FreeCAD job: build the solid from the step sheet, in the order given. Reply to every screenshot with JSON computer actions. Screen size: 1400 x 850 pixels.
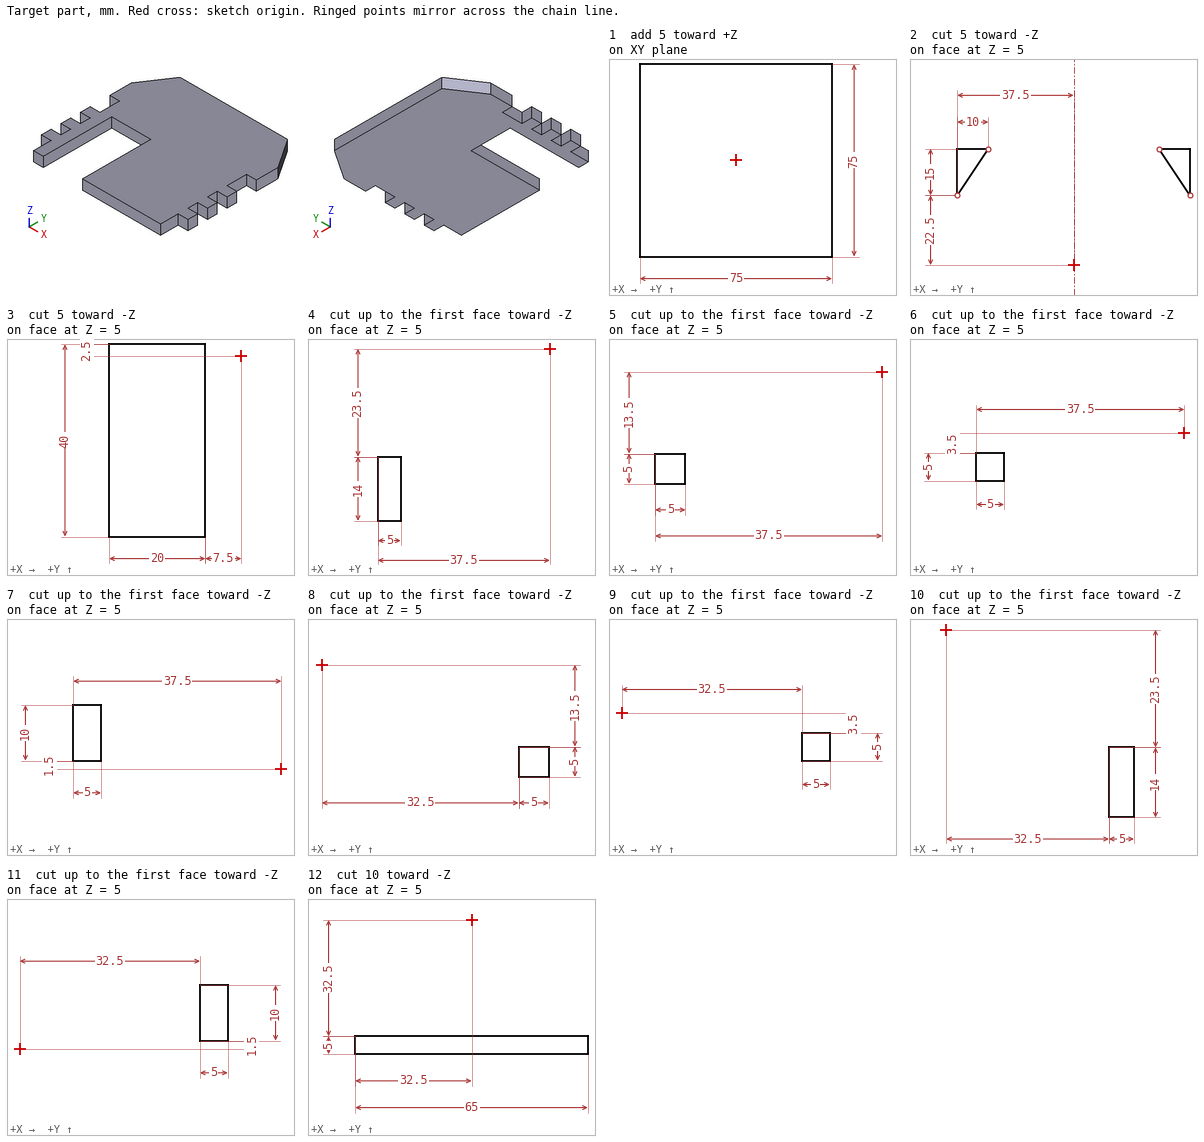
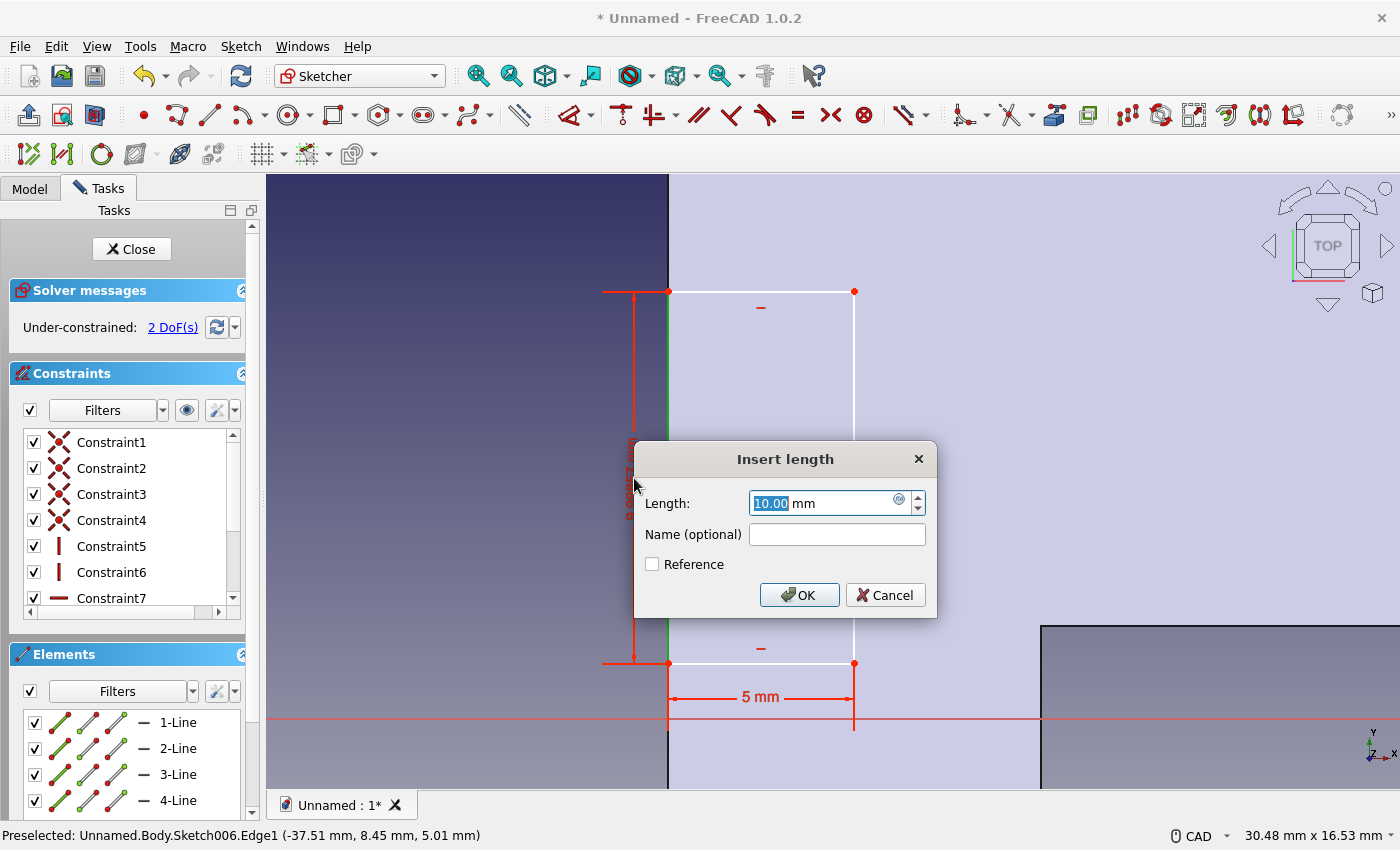
{"action": "type", "text": "10"}
{"action": "key", "text": "Return"}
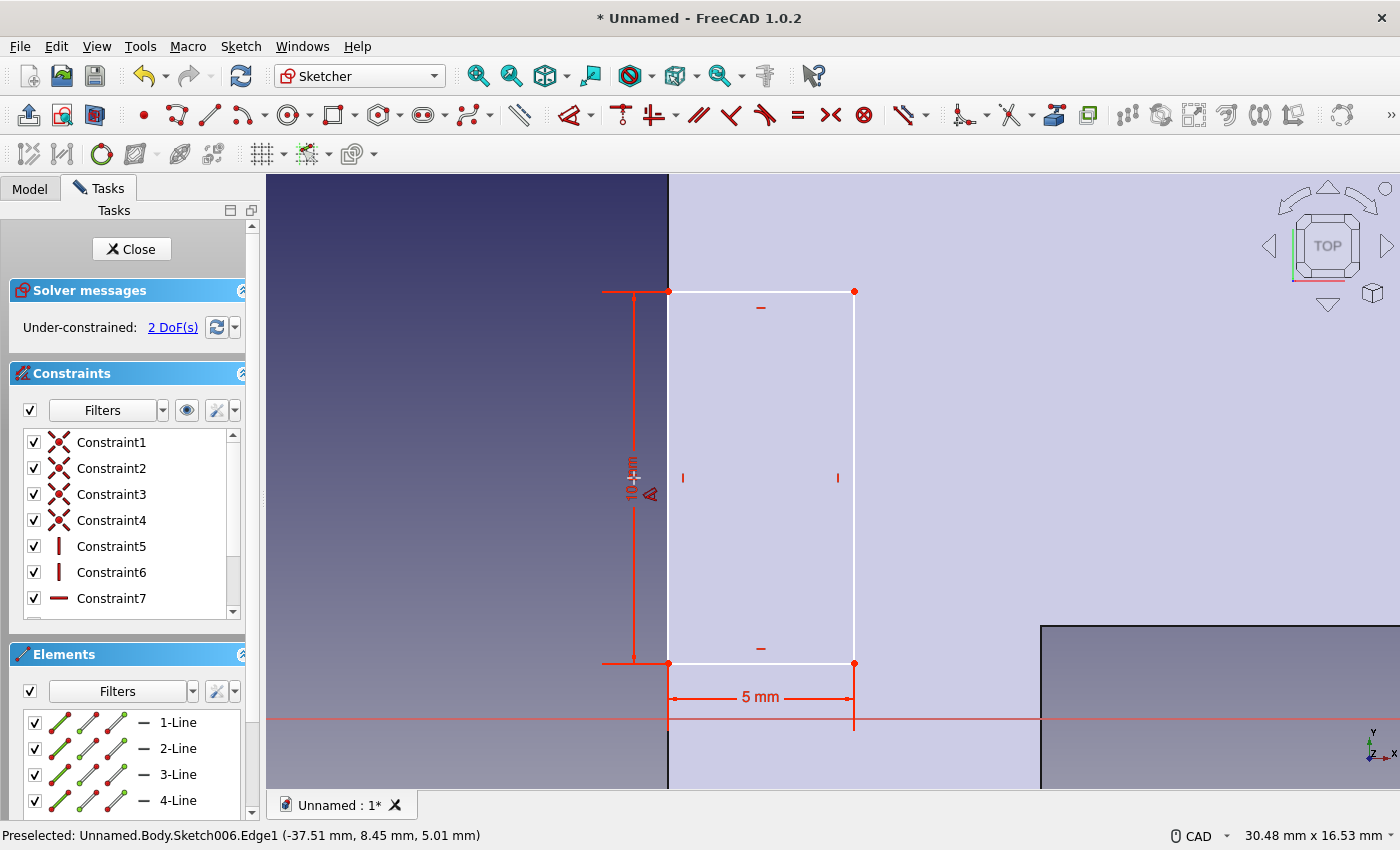
{"action": "left_click", "coordinate": [668, 664]}
{"action": "left_click", "coordinate": [634, 692]}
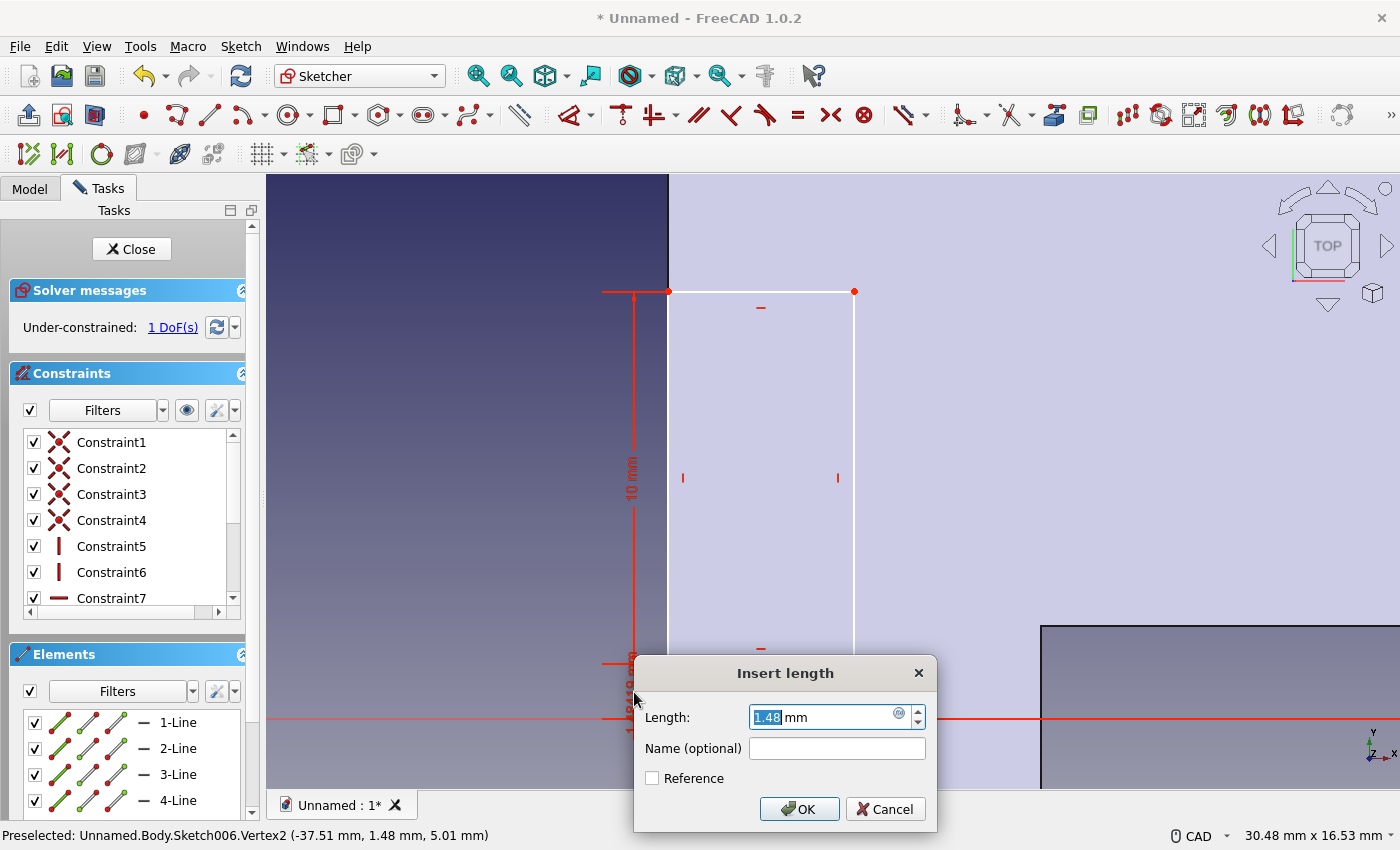
{"action": "type", "text": "1.5"}
{"action": "key", "text": "Return"}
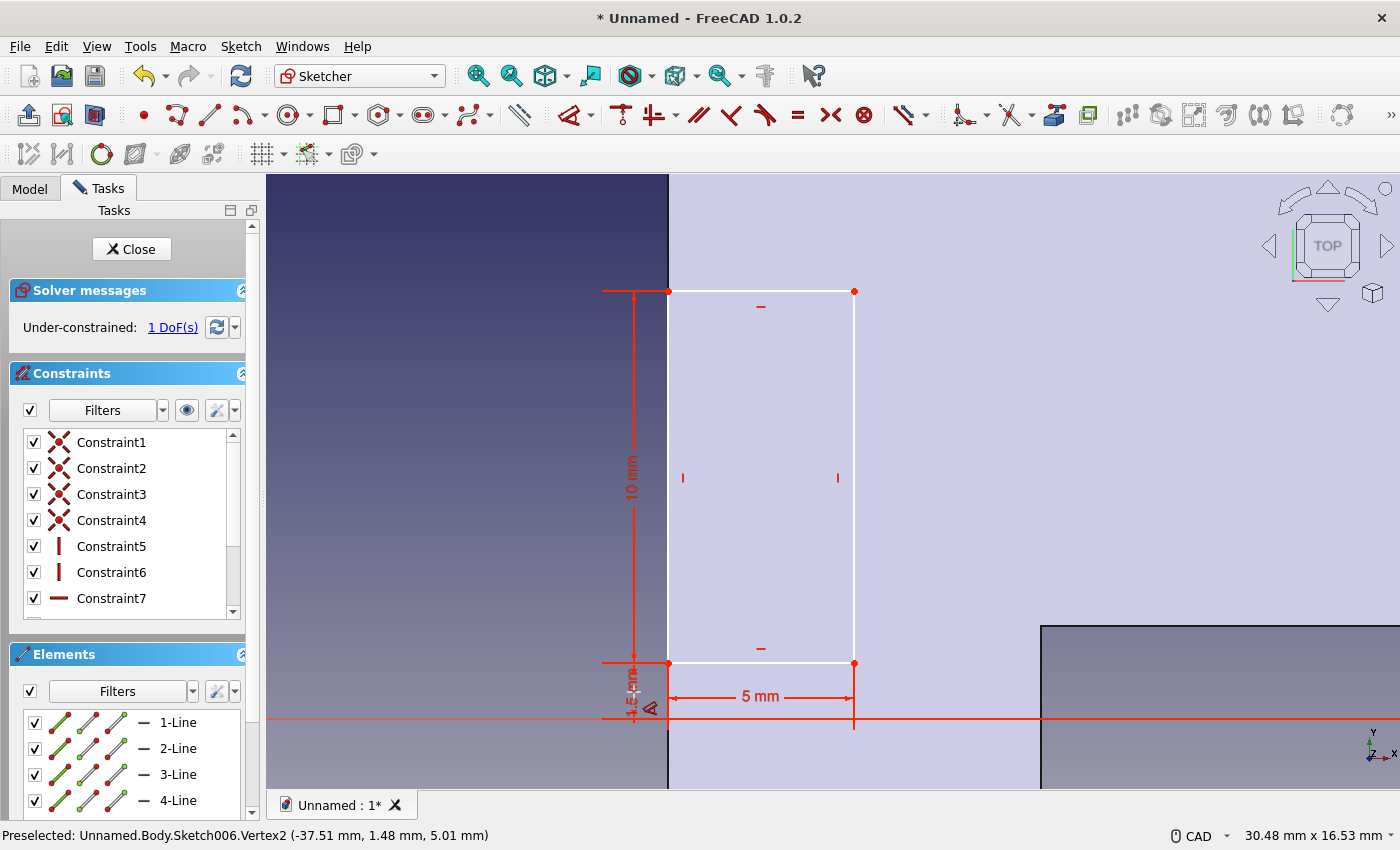
{"action": "left_click", "coordinate": [668, 291]}
{"action": "left_click", "coordinate": [952, 753]}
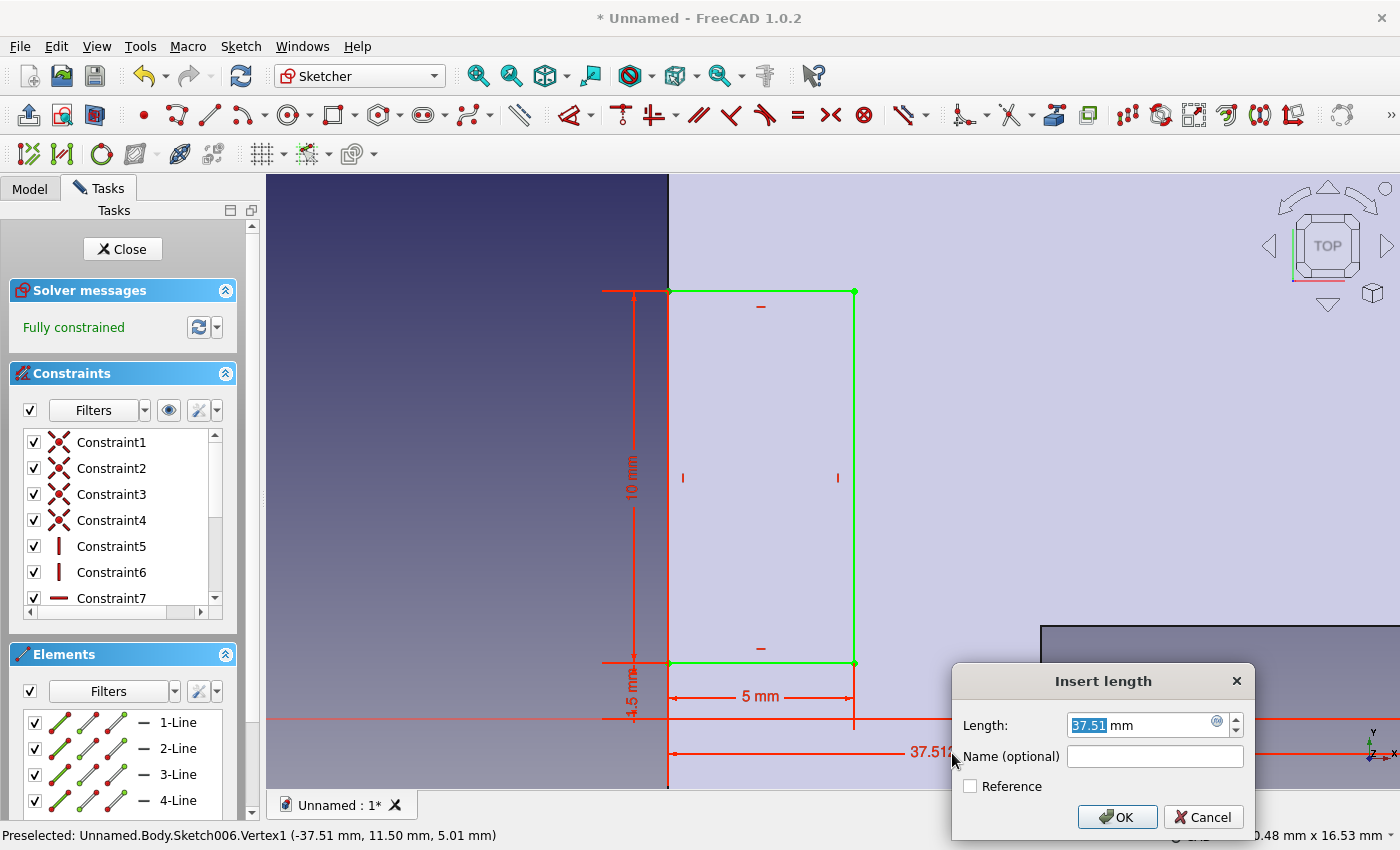
{"action": "type", "text": "37.5"}
{"action": "key", "text": "Return"}
{"action": "key", "text": "Escape"}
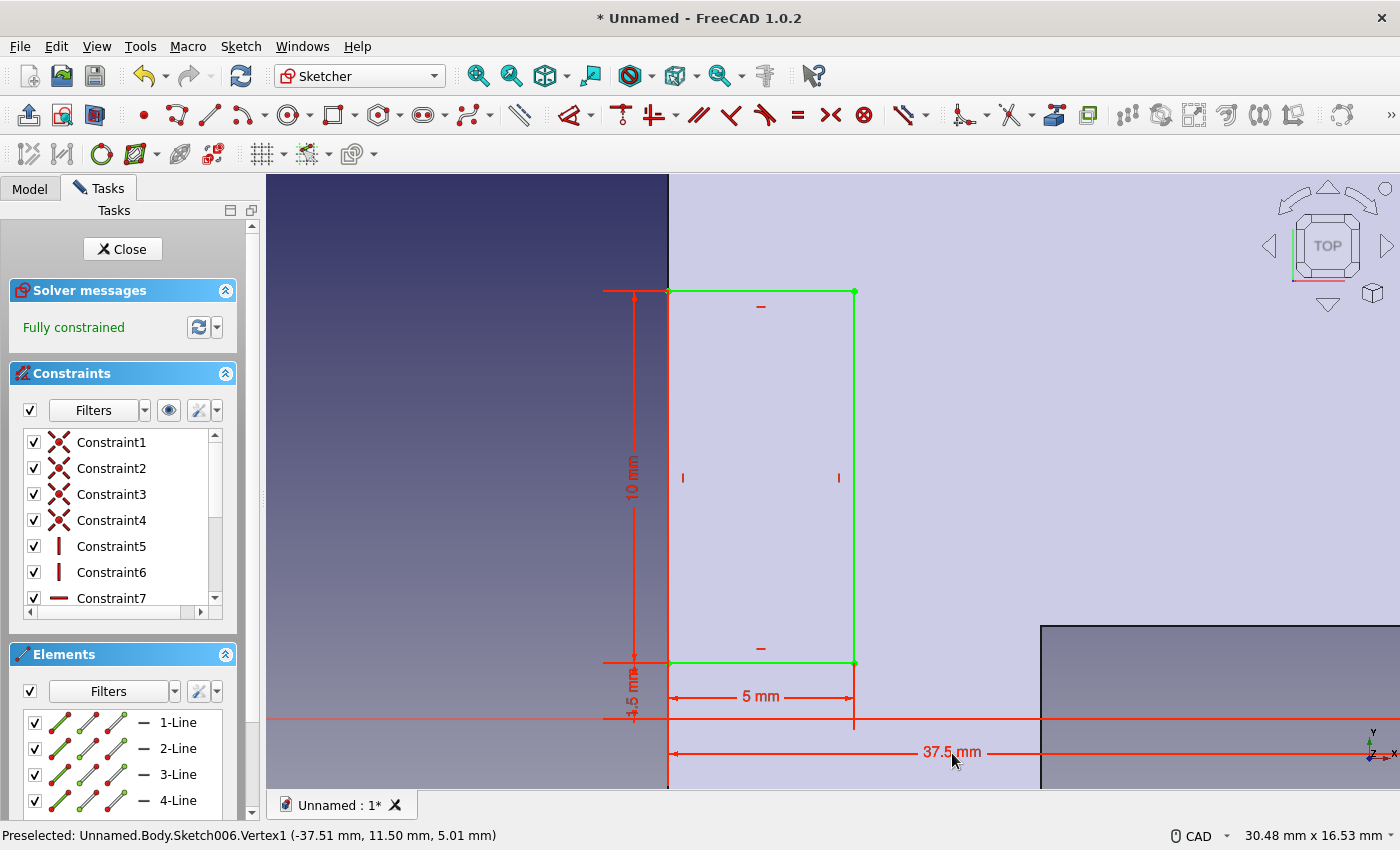
{"action": "left_click", "coordinate": [123, 249]}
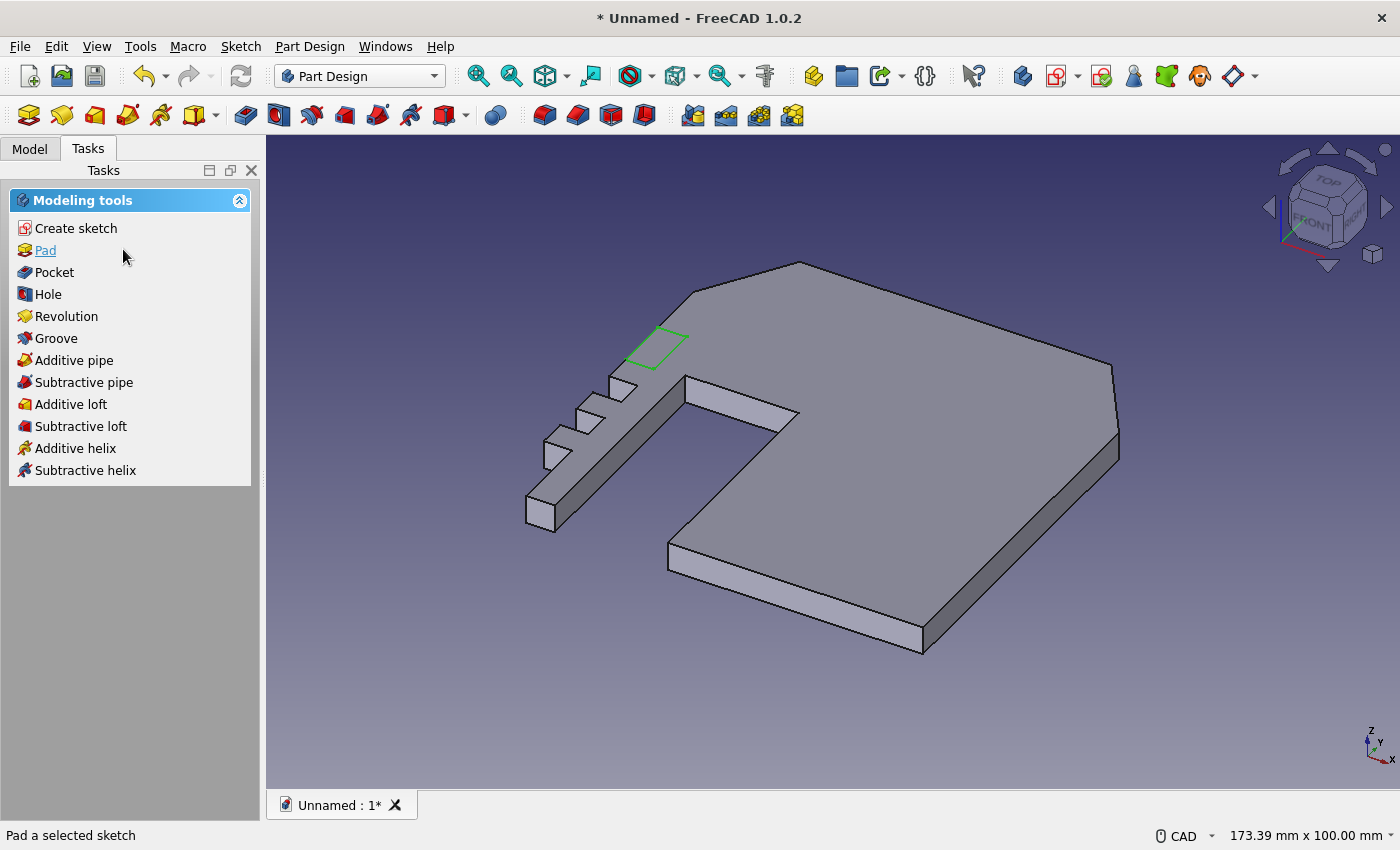
{"action": "left_click", "coordinate": [246, 116]}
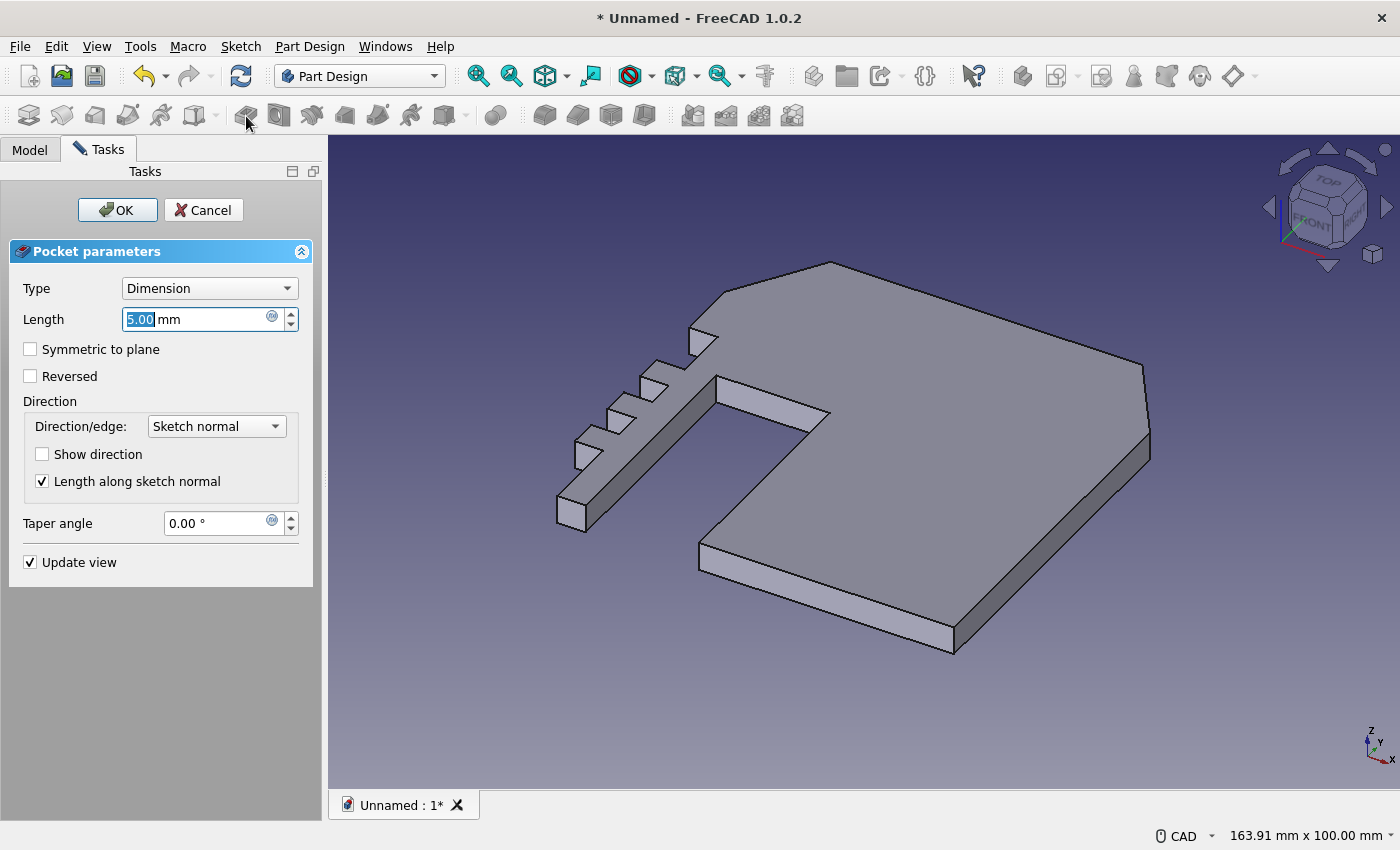
{"action": "left_click", "coordinate": [210, 288]}